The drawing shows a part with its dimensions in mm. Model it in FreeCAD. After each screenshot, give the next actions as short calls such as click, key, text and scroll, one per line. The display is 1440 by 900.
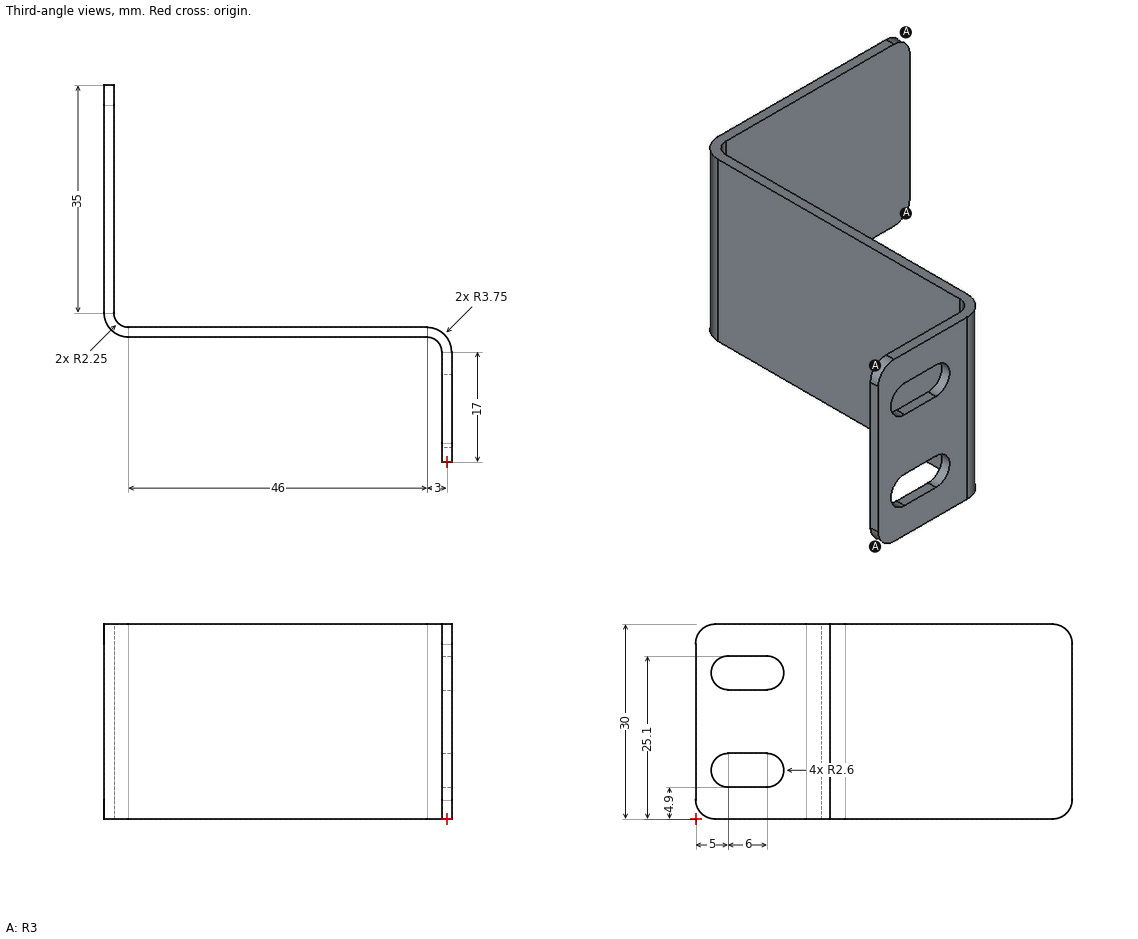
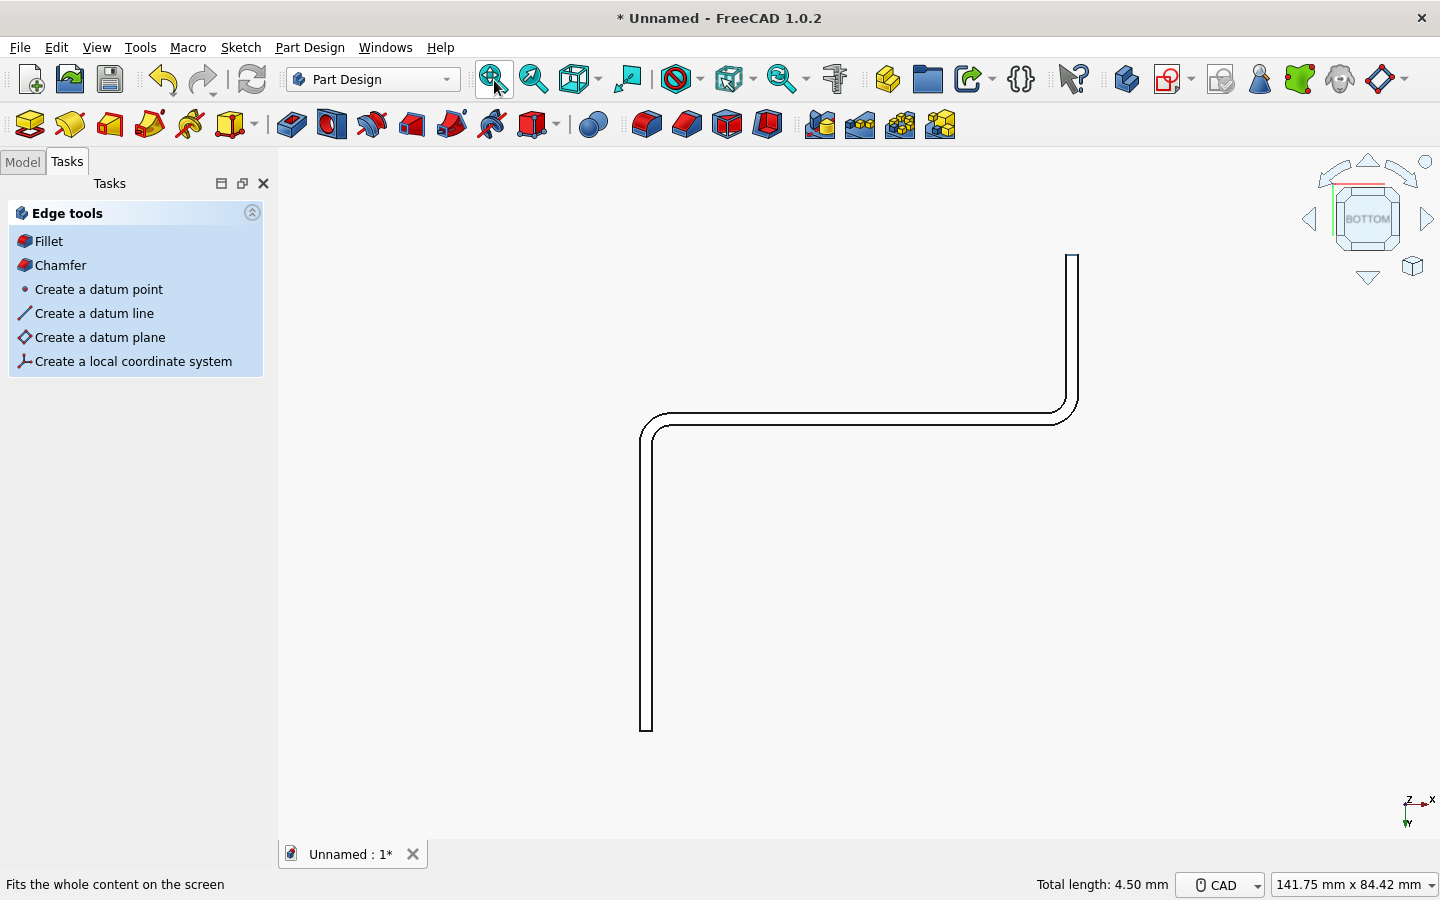
click(646, 730, ctrl)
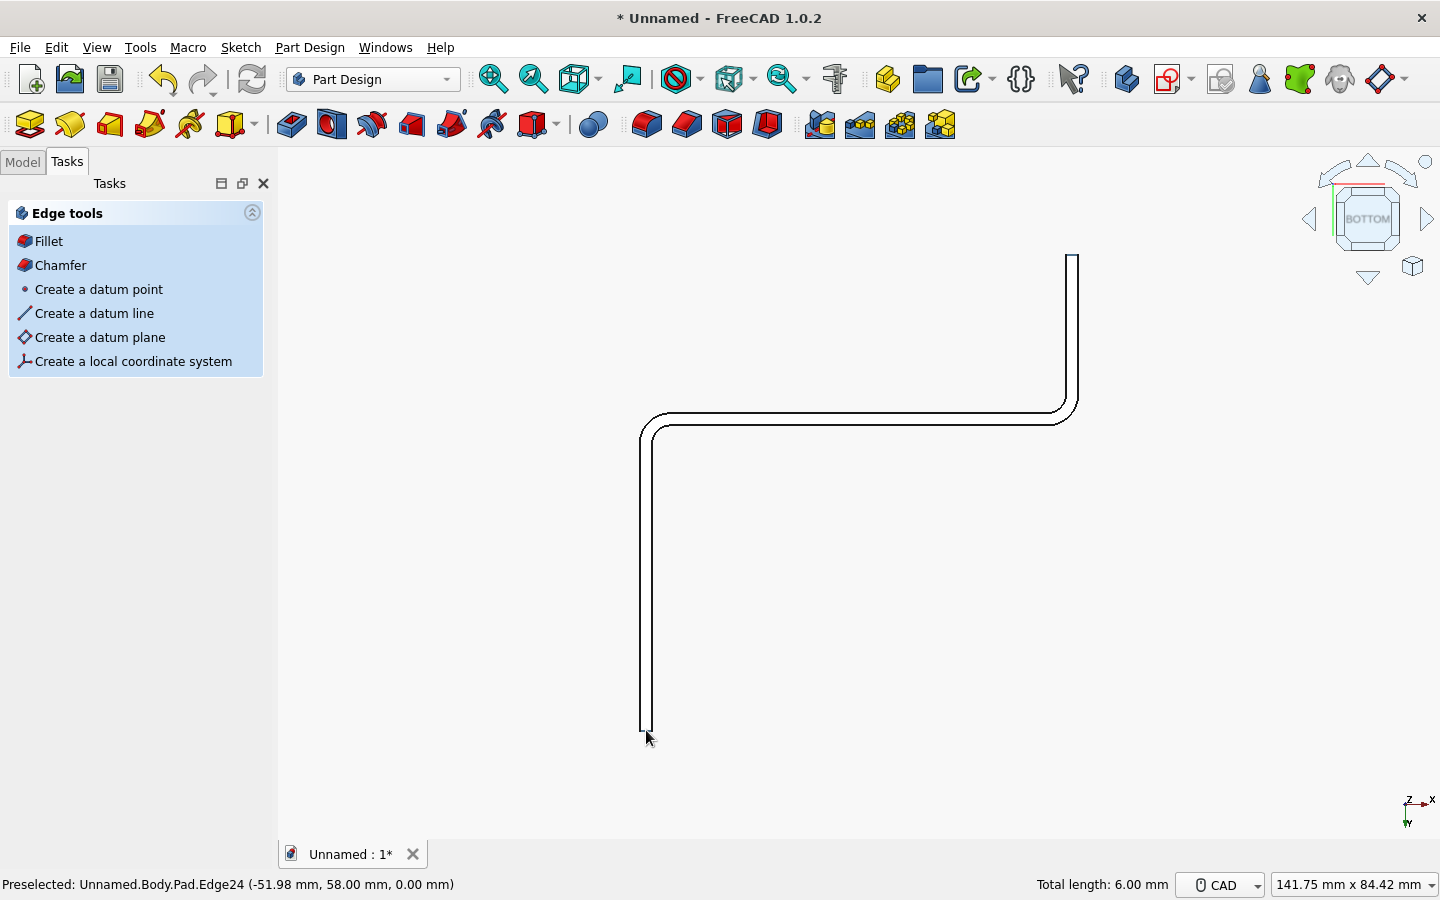
click(648, 124)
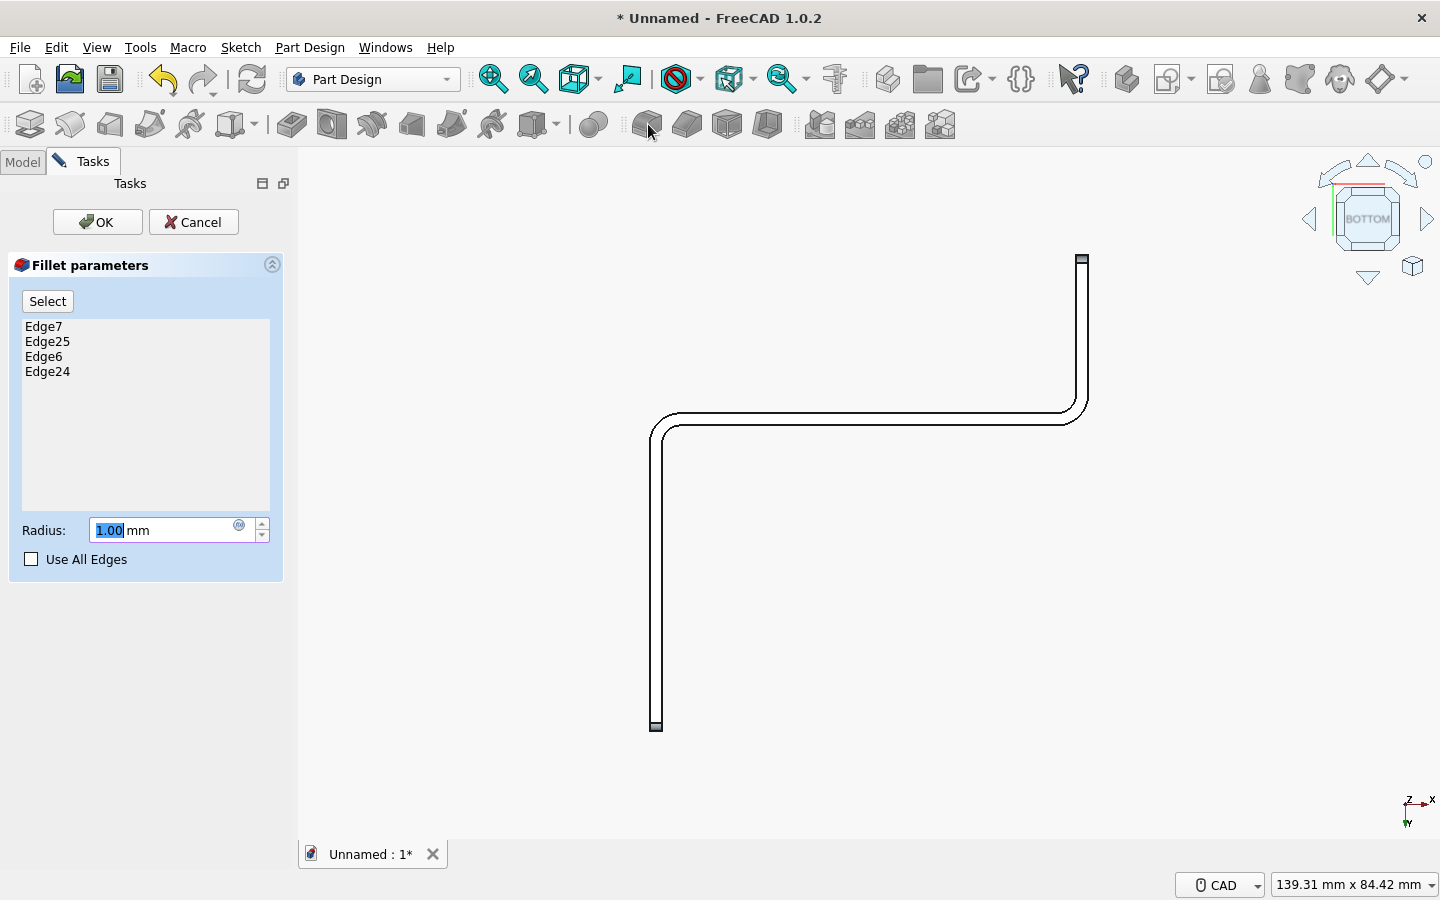
text(3)
key(Tab)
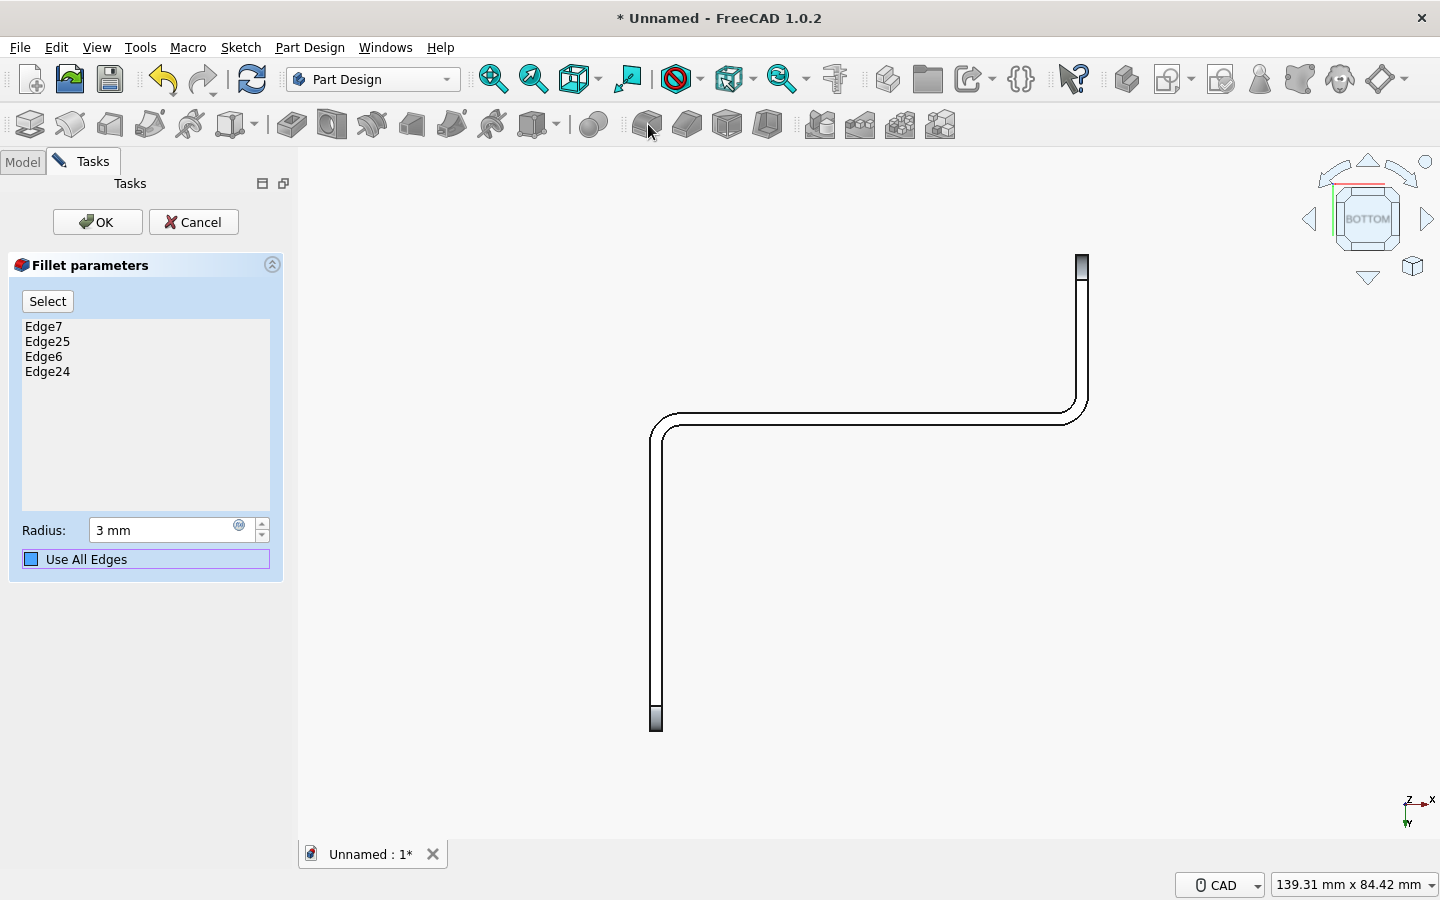
click(98, 222)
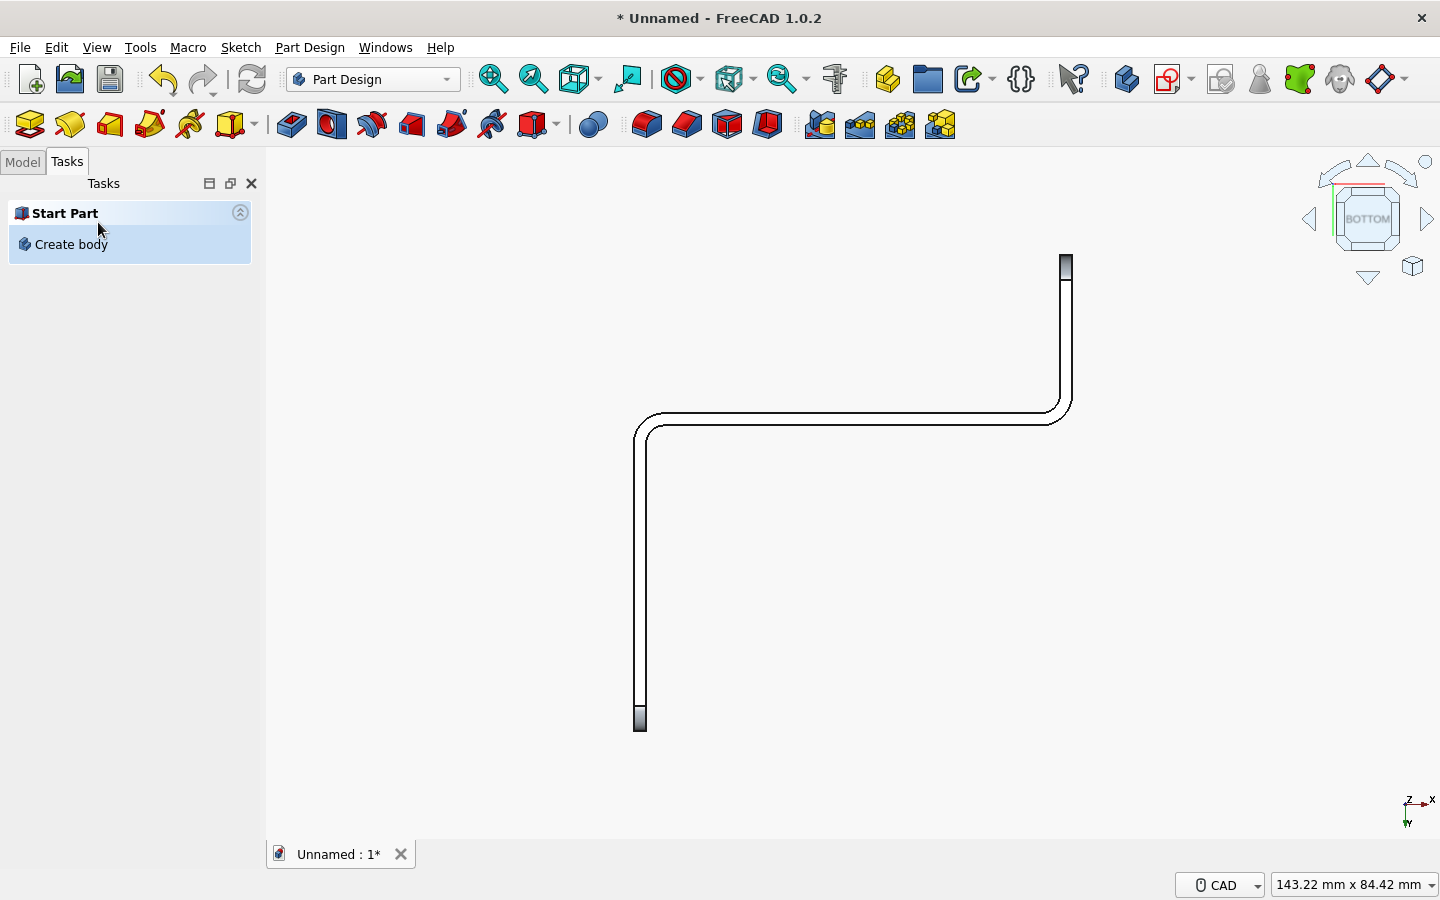
key(6)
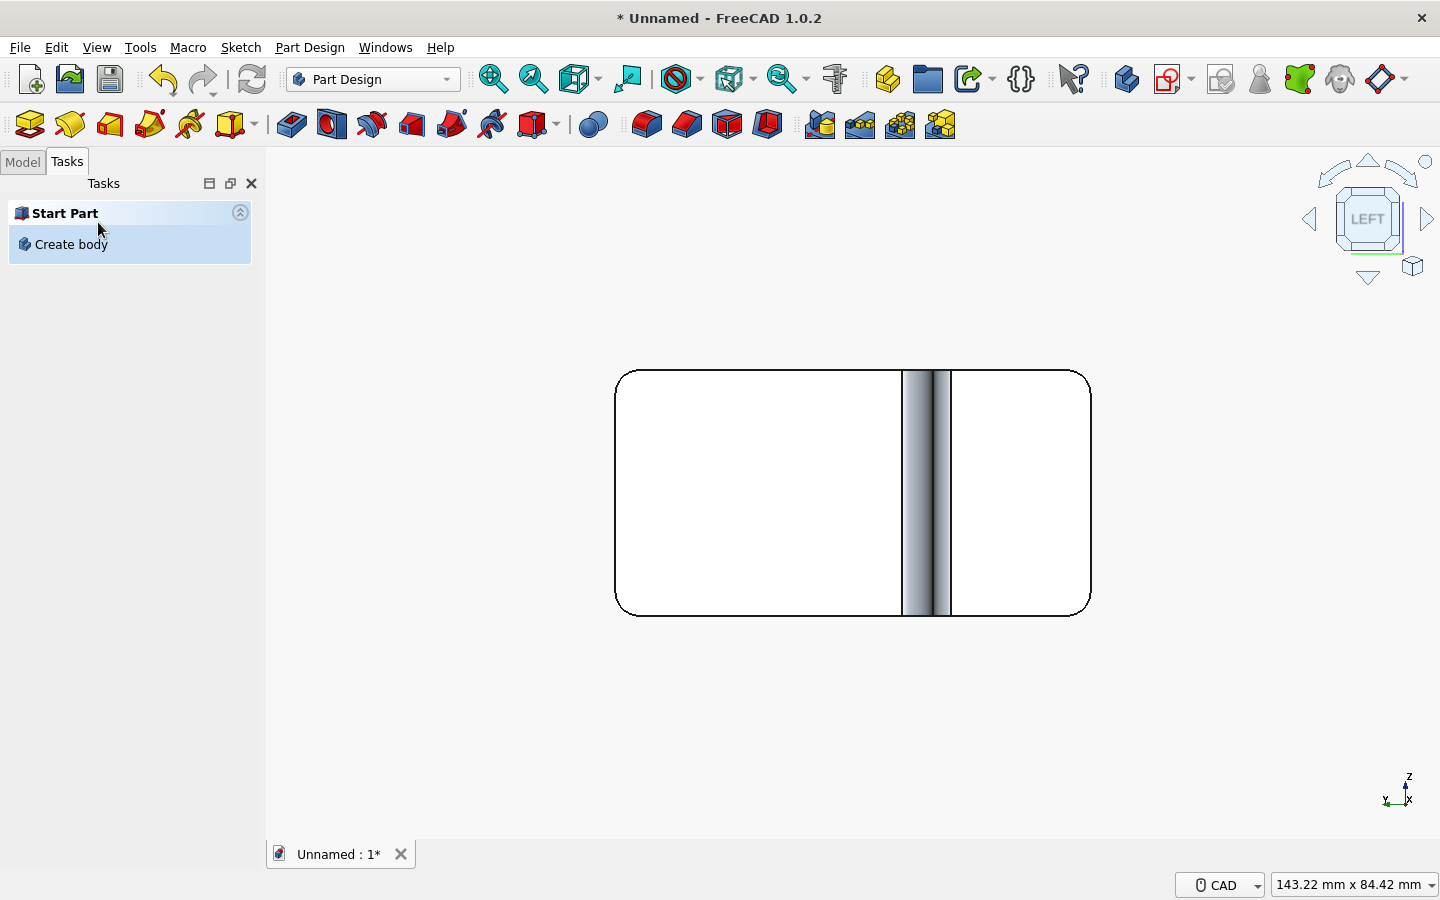
key(v)
key(f)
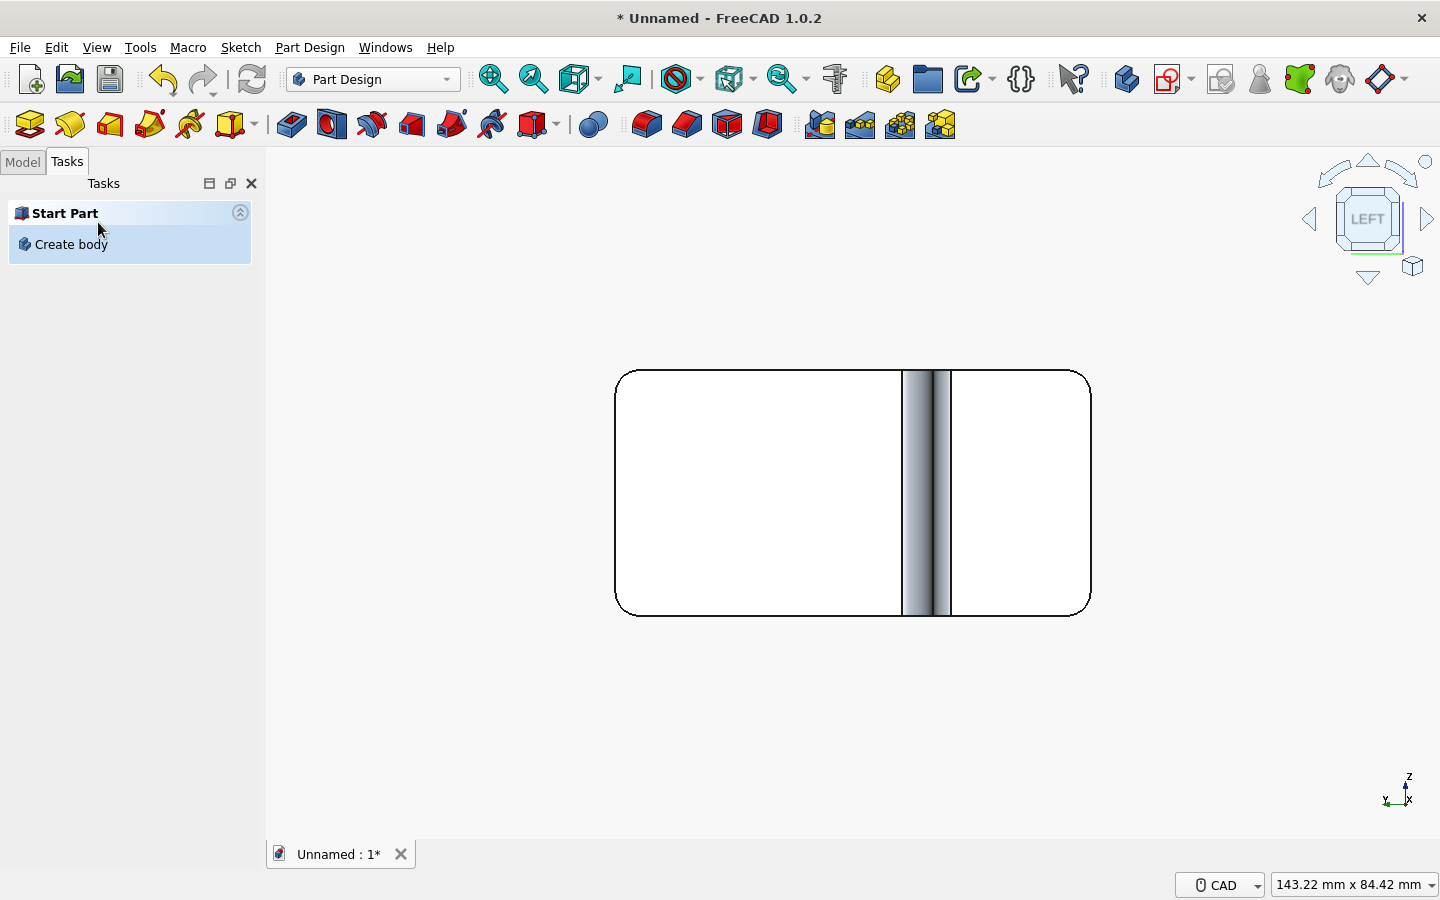
click(1021, 457)